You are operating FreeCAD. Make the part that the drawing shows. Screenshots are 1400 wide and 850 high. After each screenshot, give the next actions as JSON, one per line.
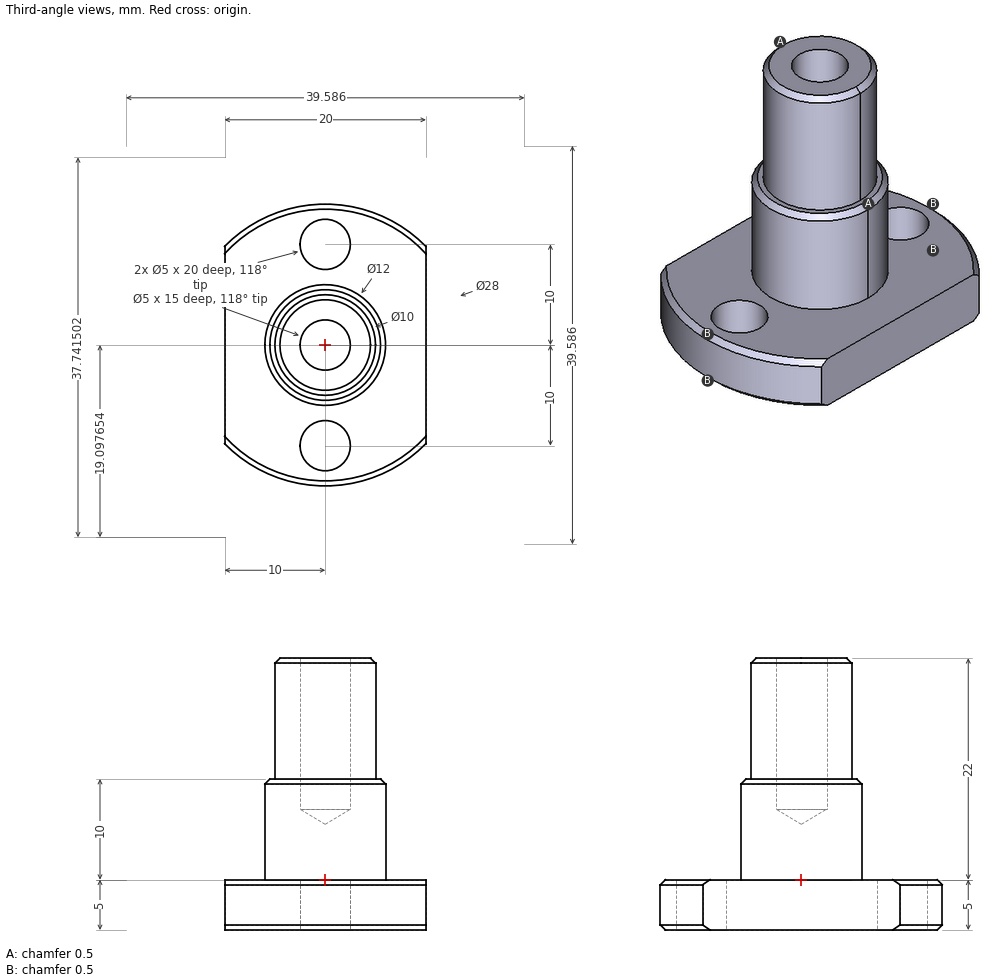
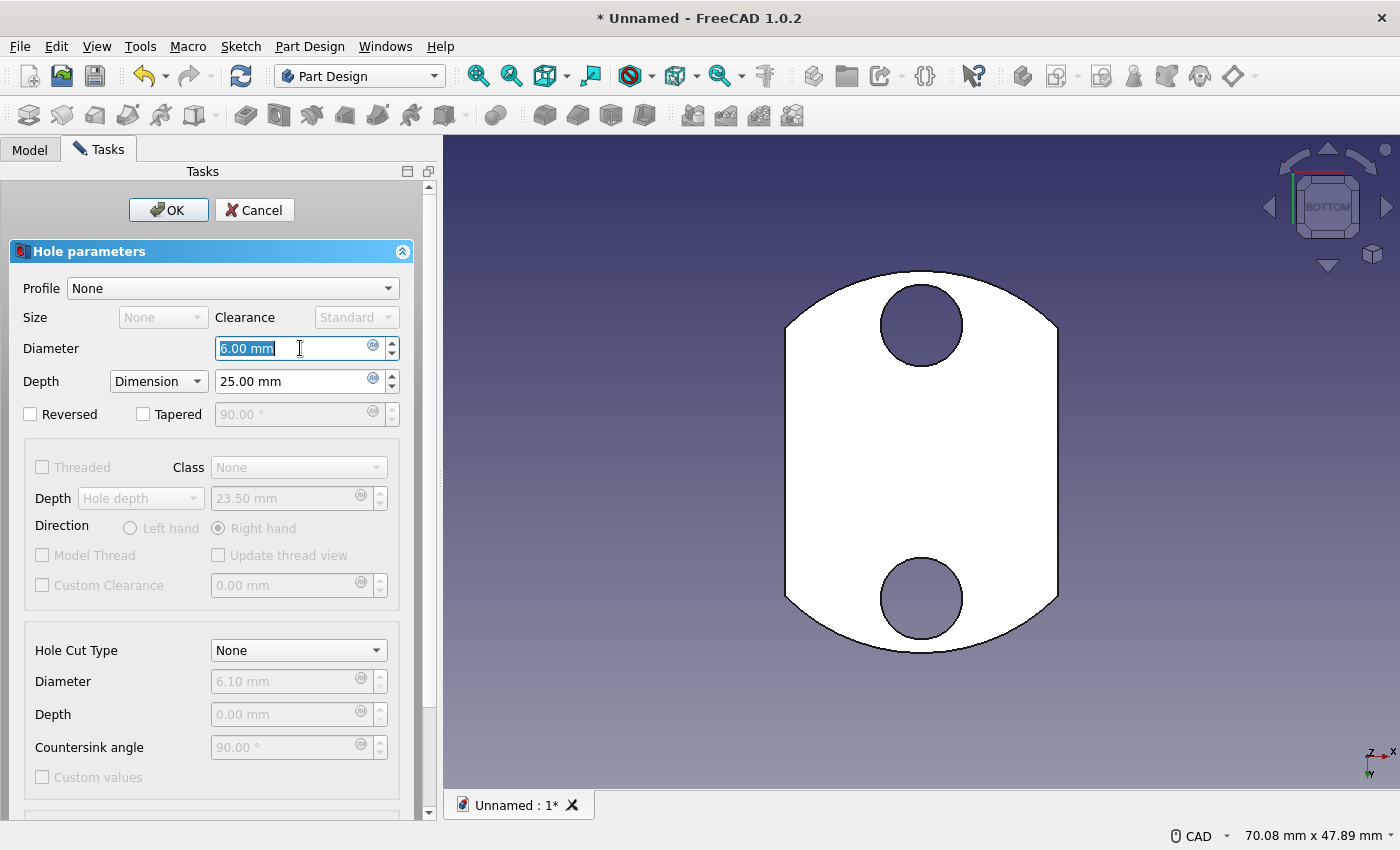
{"action": "type", "text": "5"}
{"action": "key", "text": "Tab"}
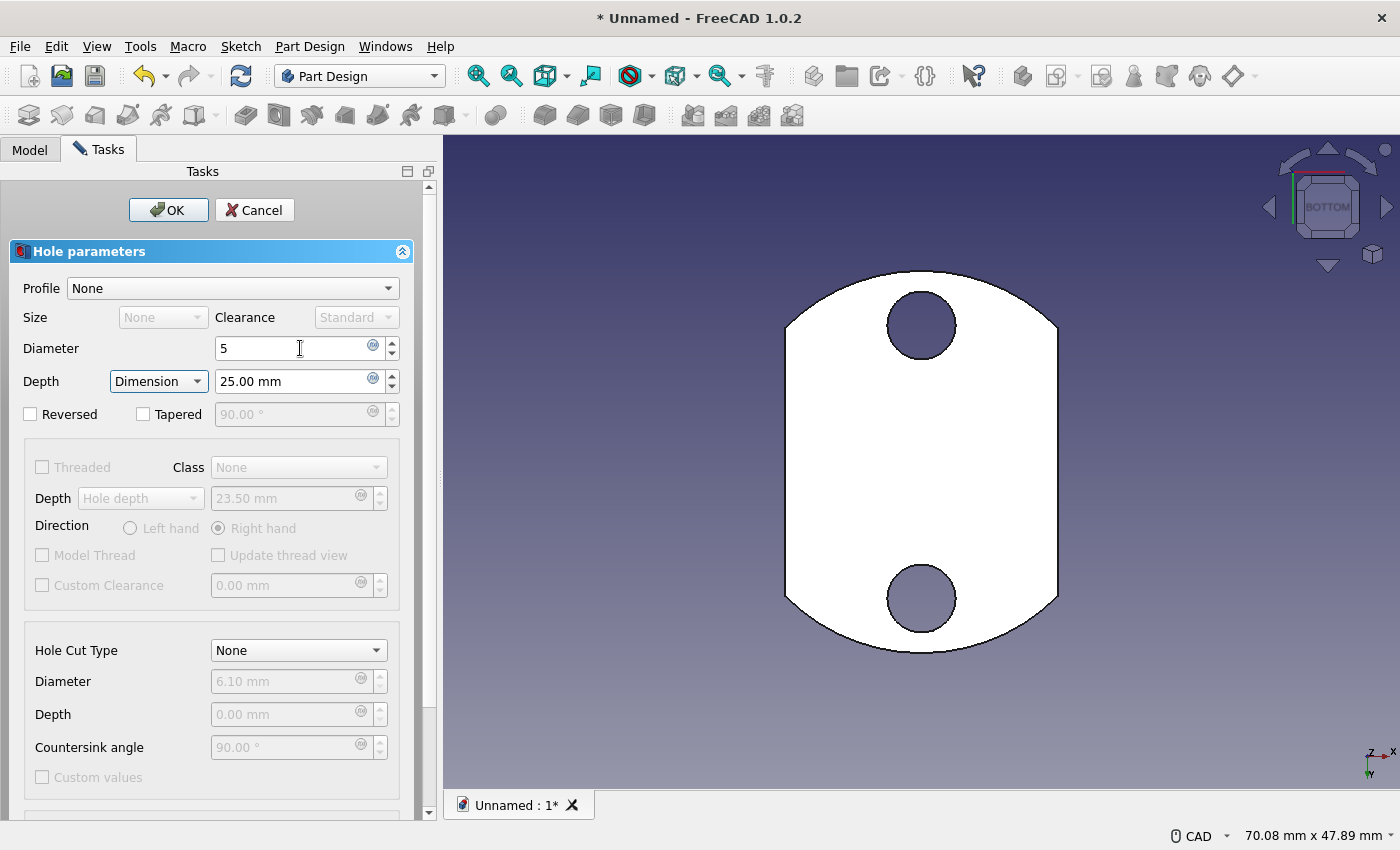
{"action": "triple_click", "coordinate": [300, 382]}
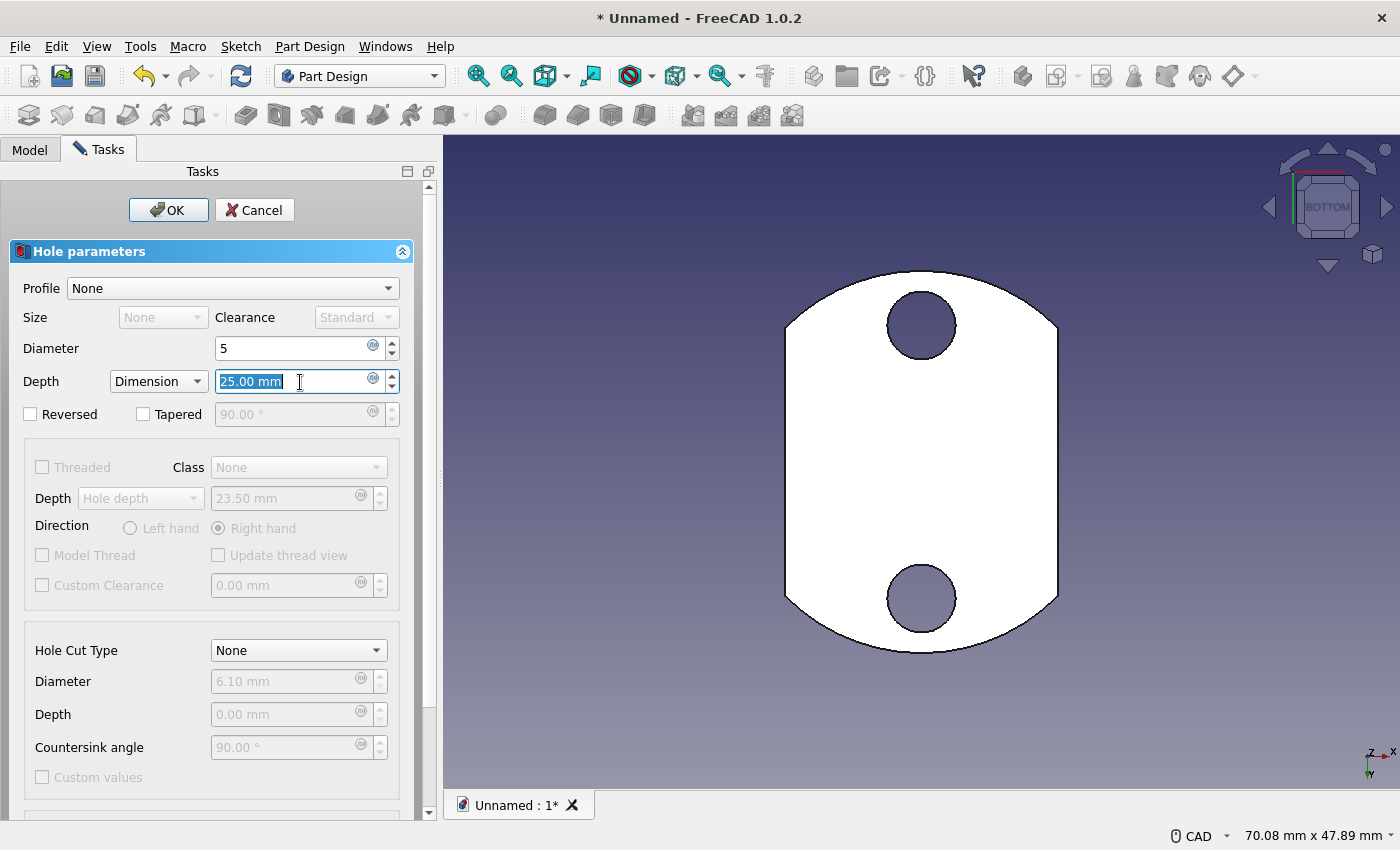
{"action": "type", "text": "20"}
{"action": "key", "text": "Tab"}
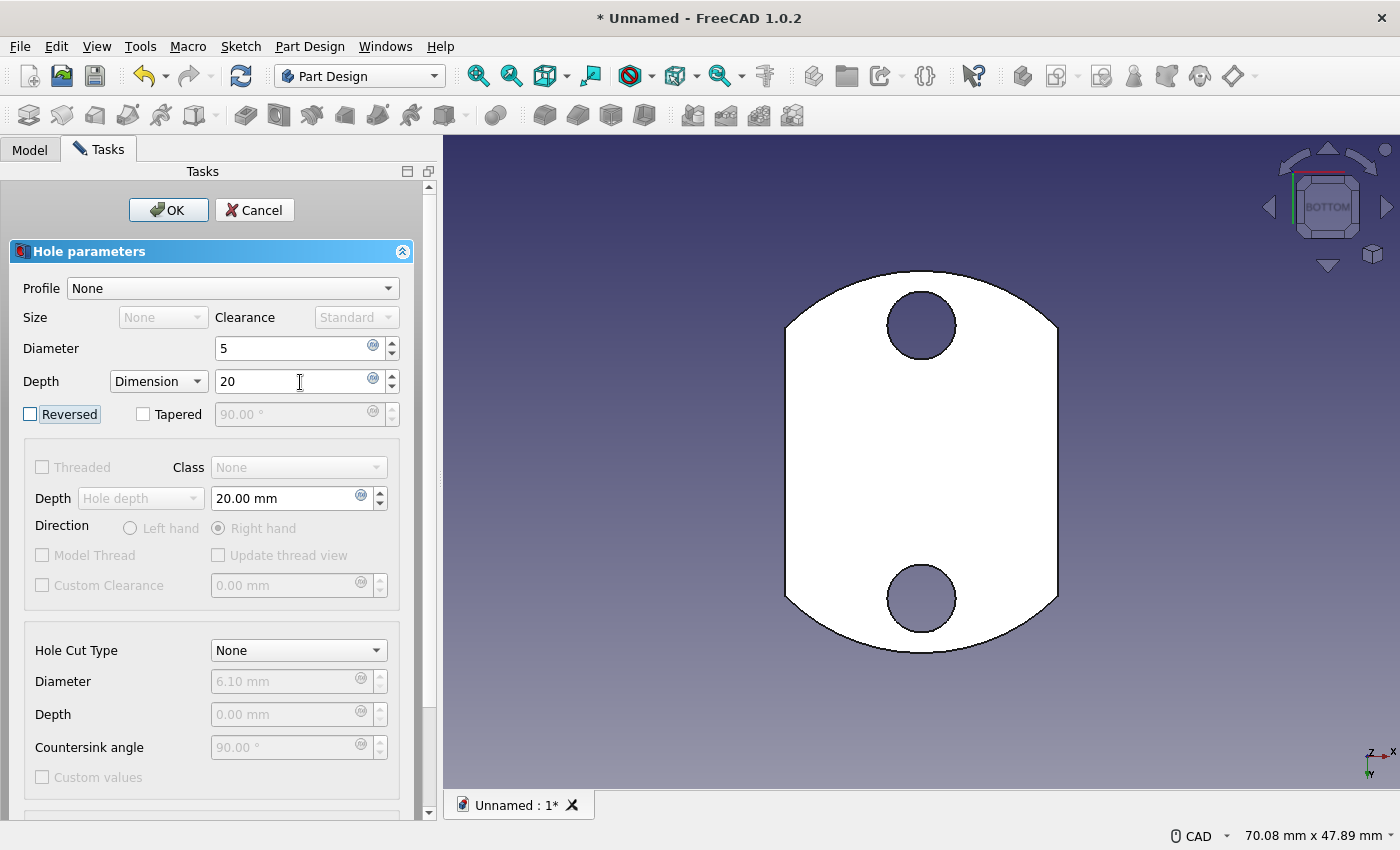
{"action": "left_click", "coordinate": [169, 210]}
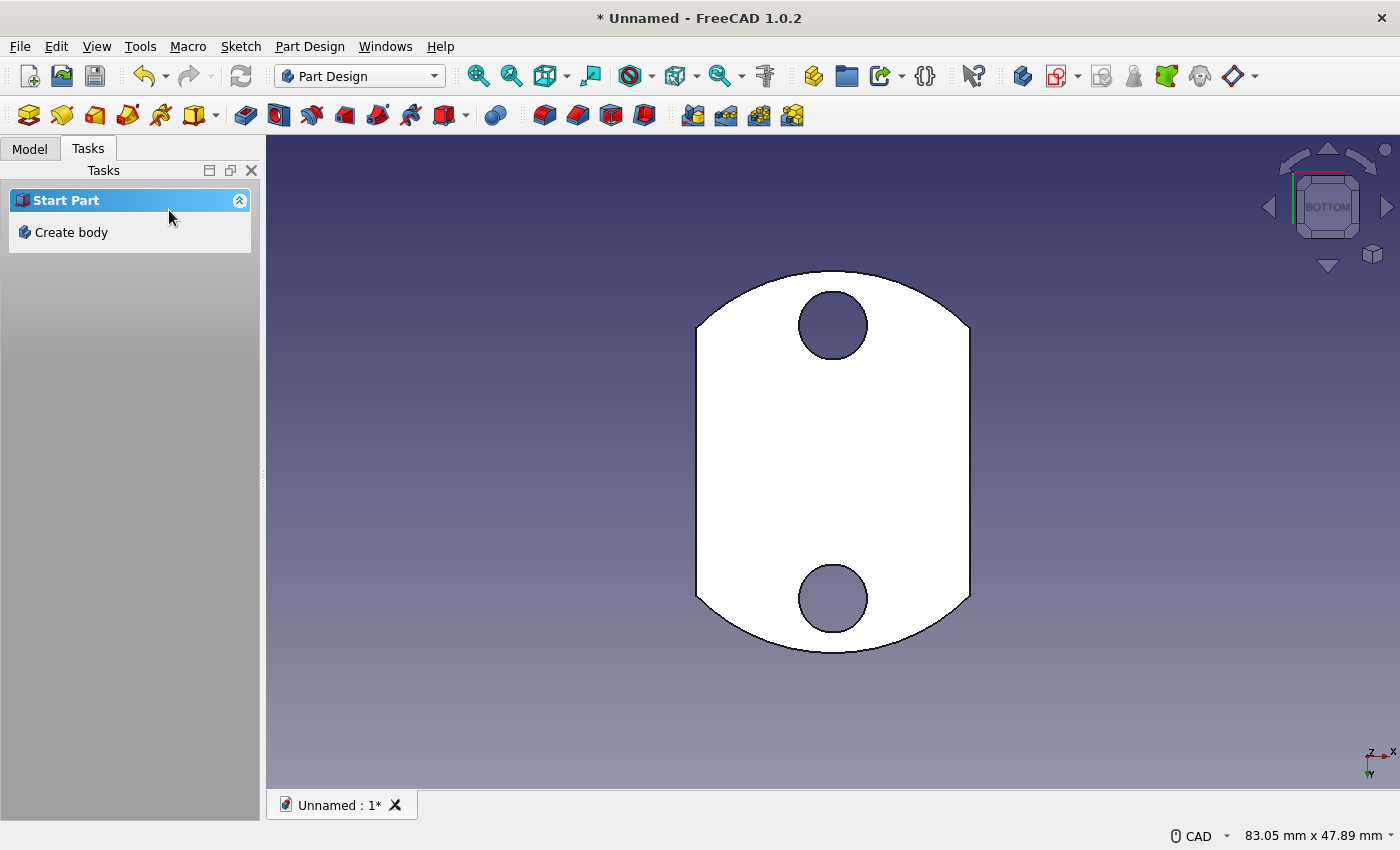
{"action": "key", "text": "0"}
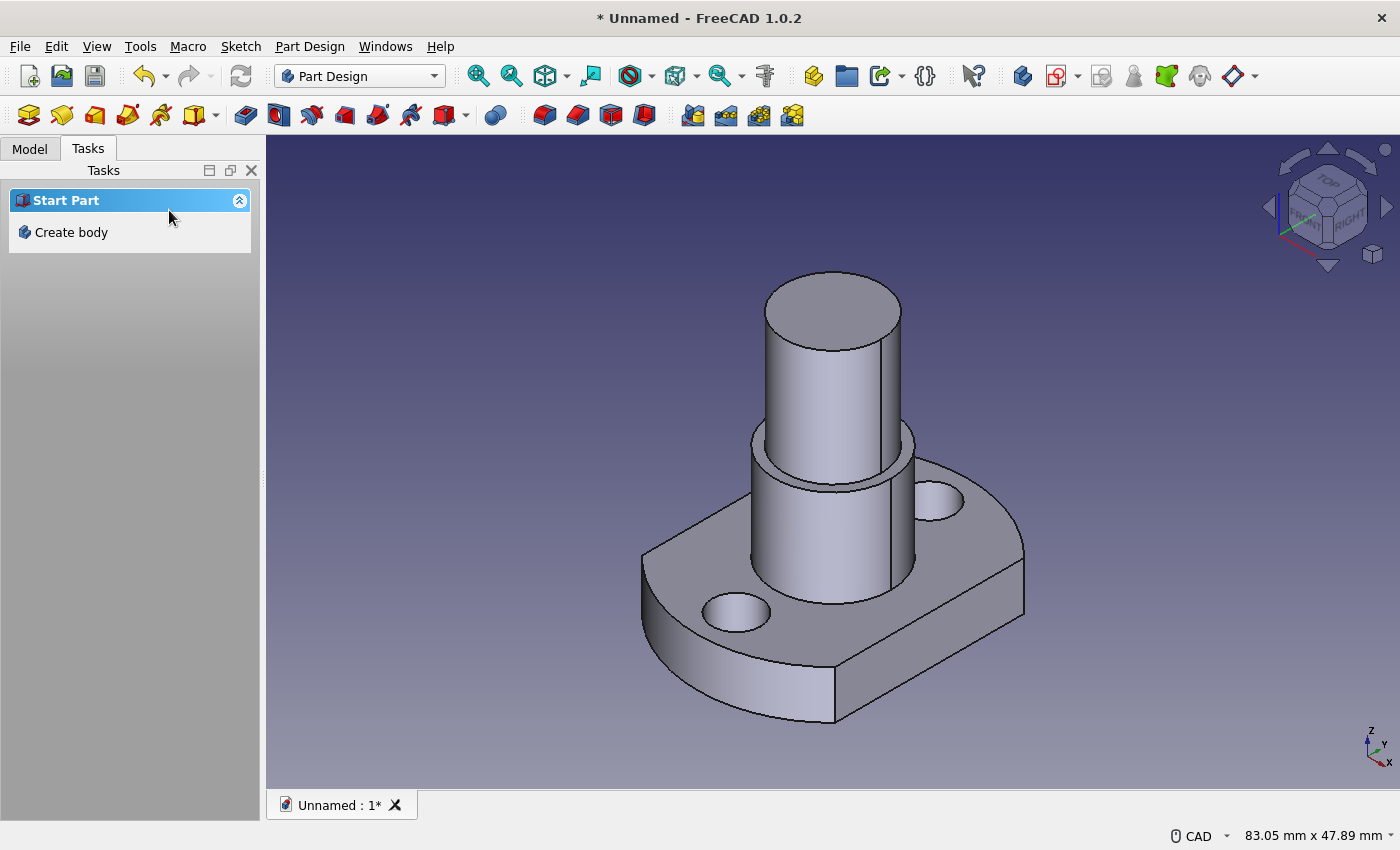
{"action": "left_click", "coordinate": [833, 310]}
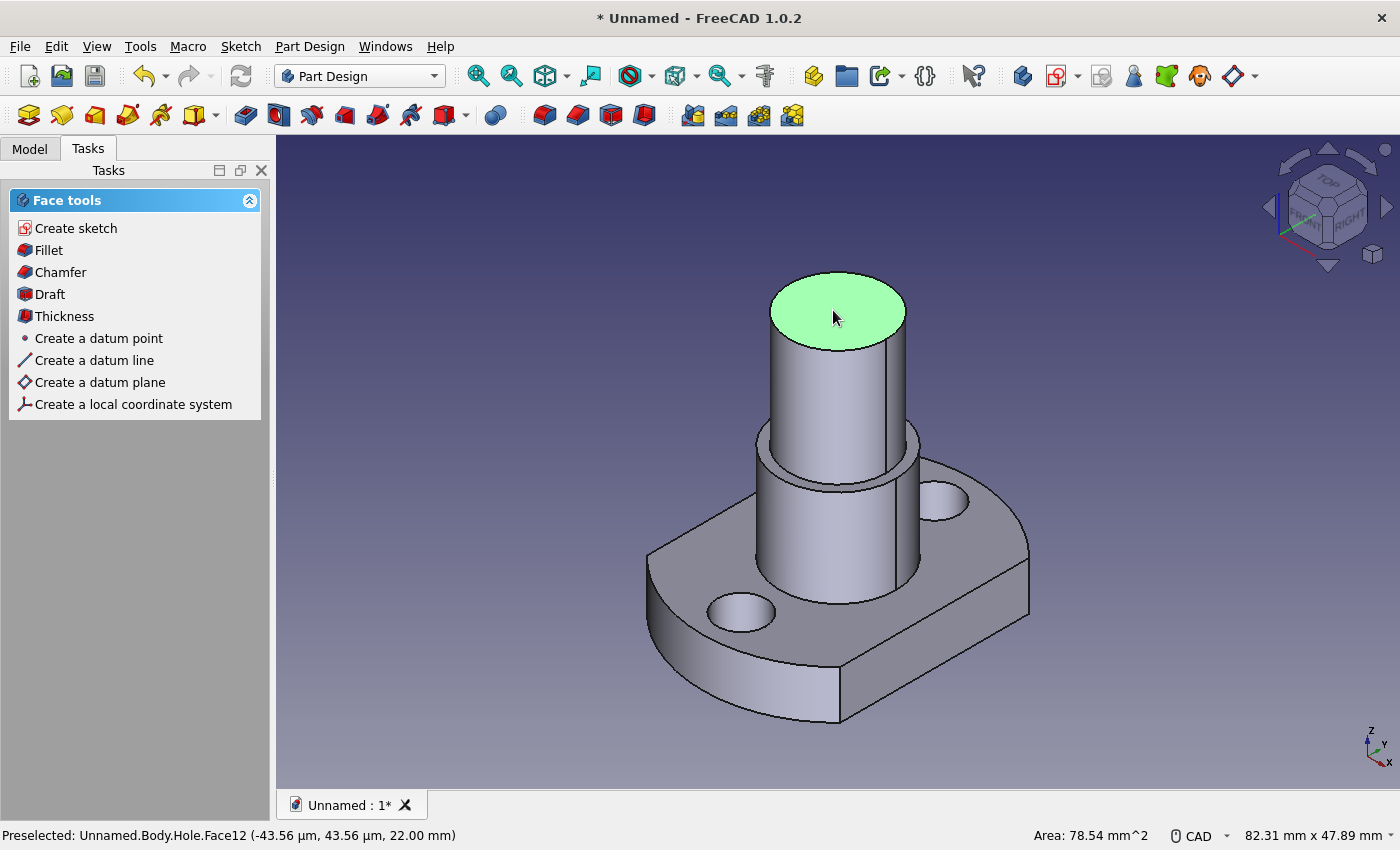
{"action": "left_click", "coordinate": [1056, 76]}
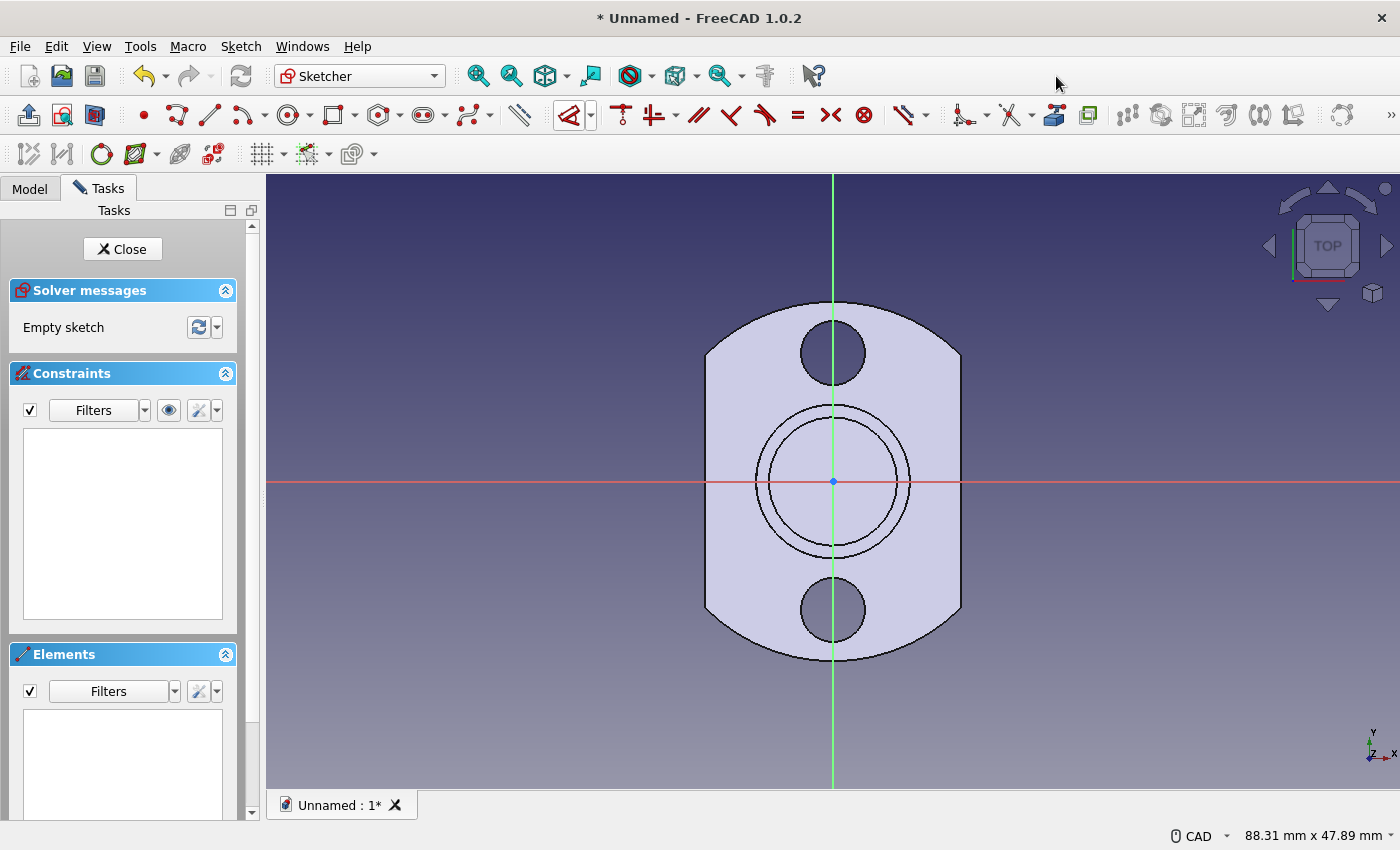
{"action": "scroll", "coordinate": [847, 481], "scroll_direction": "up", "scroll_amount": 9}